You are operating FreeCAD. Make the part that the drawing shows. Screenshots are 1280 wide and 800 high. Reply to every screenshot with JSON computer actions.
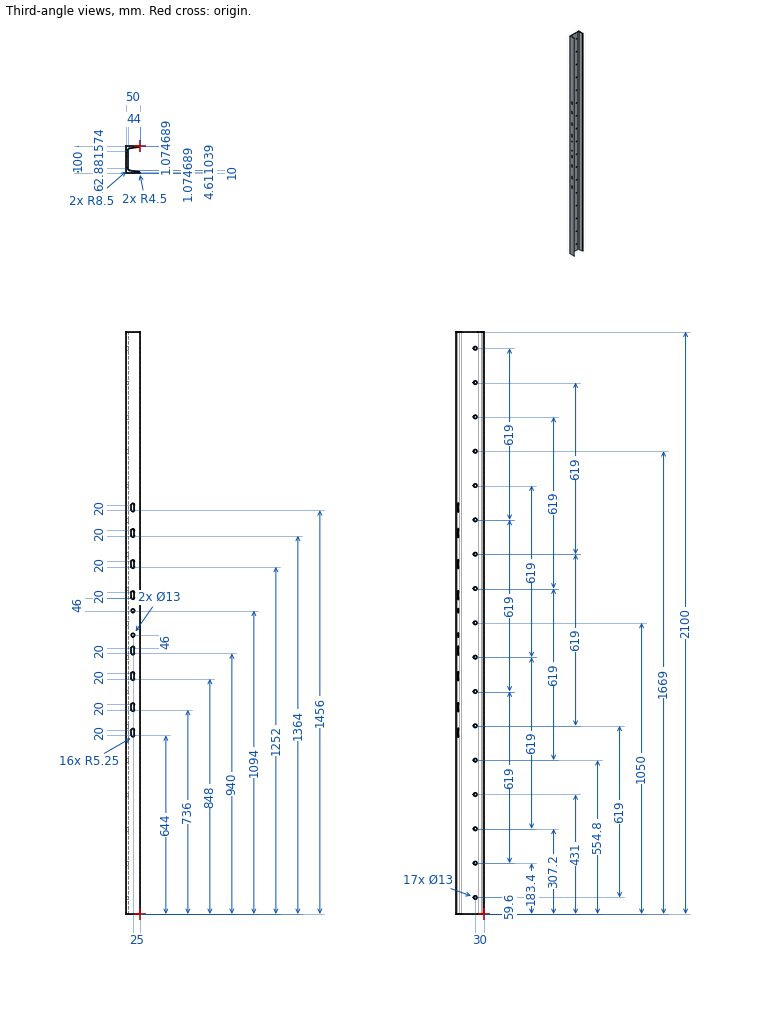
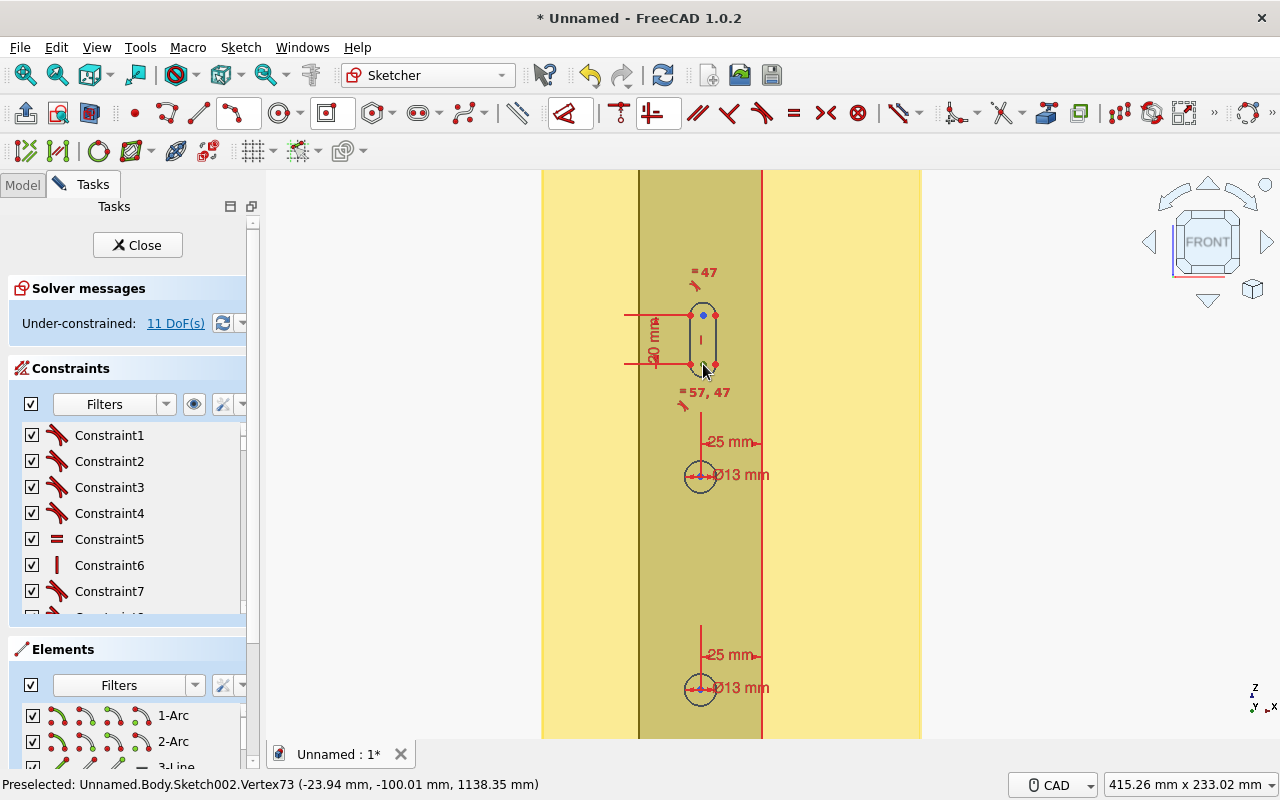
{"action": "key", "text": "l"}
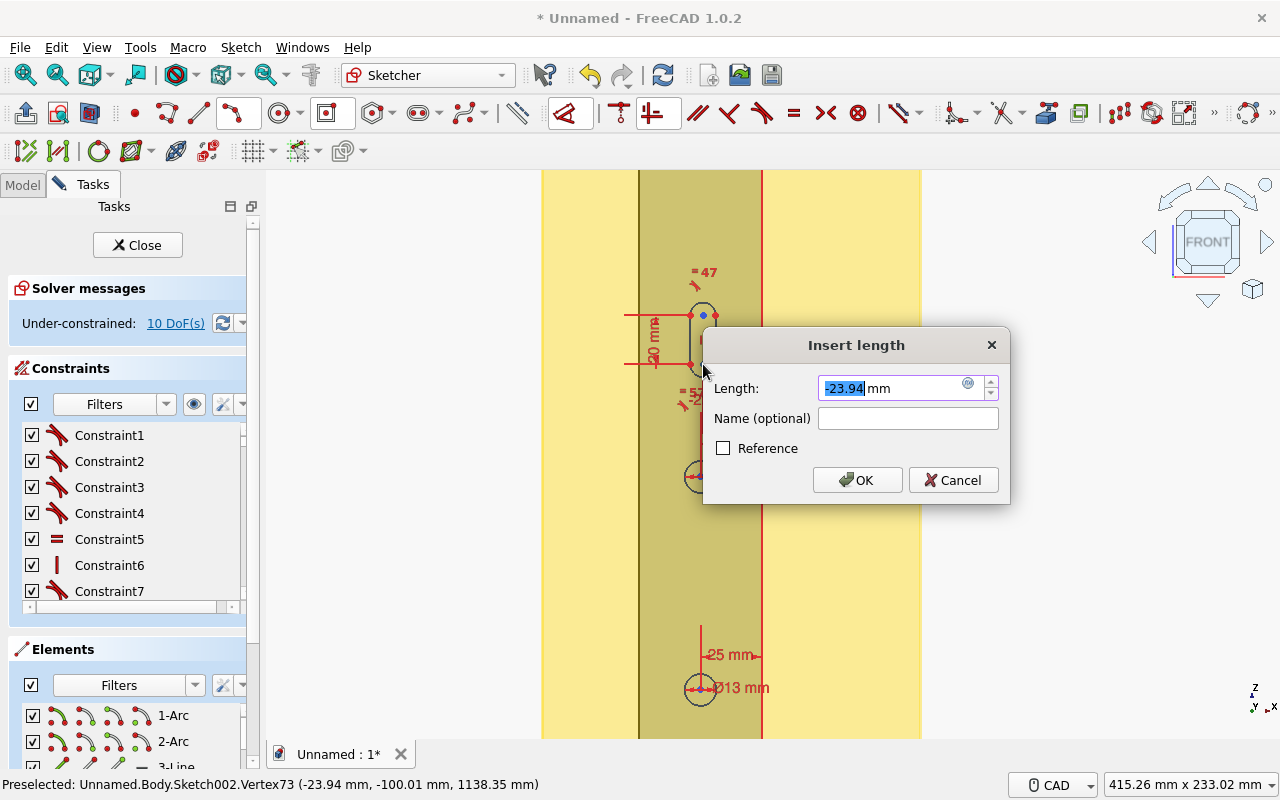
{"action": "type", "text": "-25"}
{"action": "key", "text": "Return"}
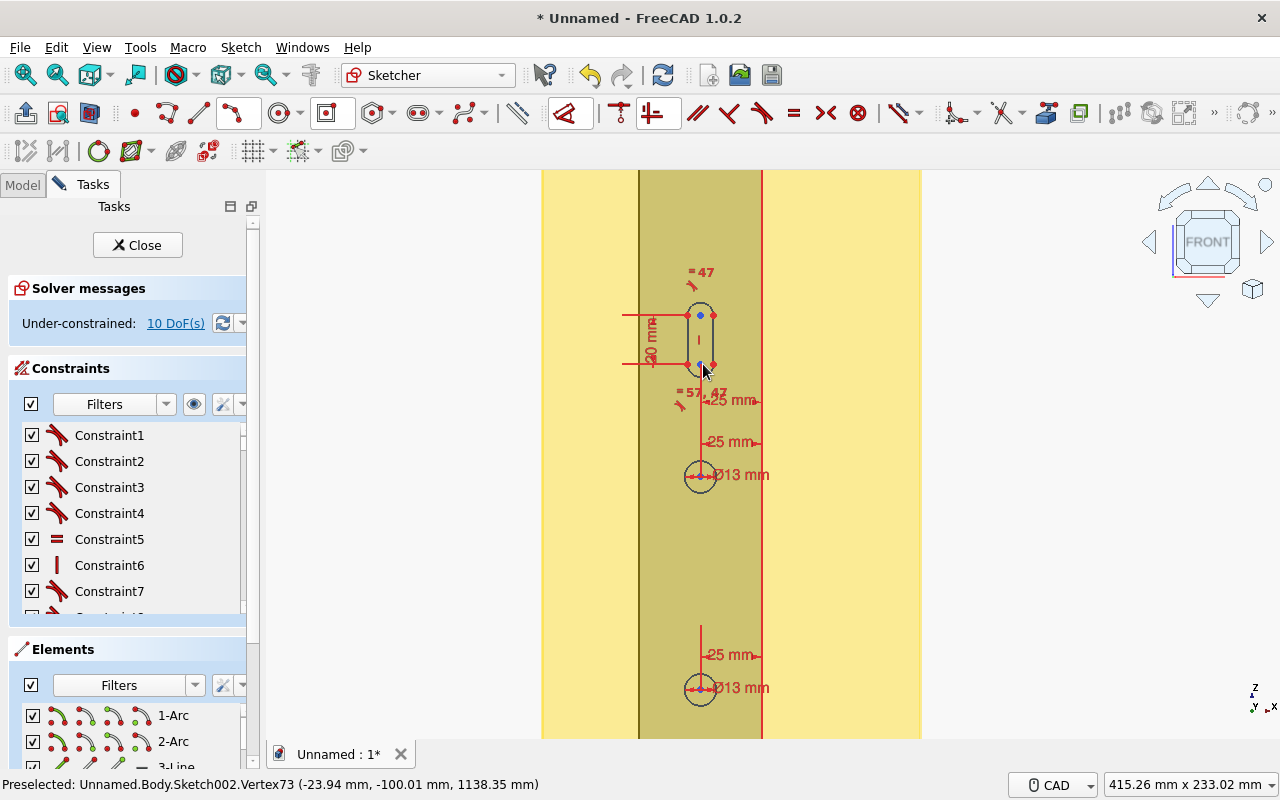
{"action": "scroll", "coordinate": [703, 367], "scroll_direction": "down", "scroll_amount": 12}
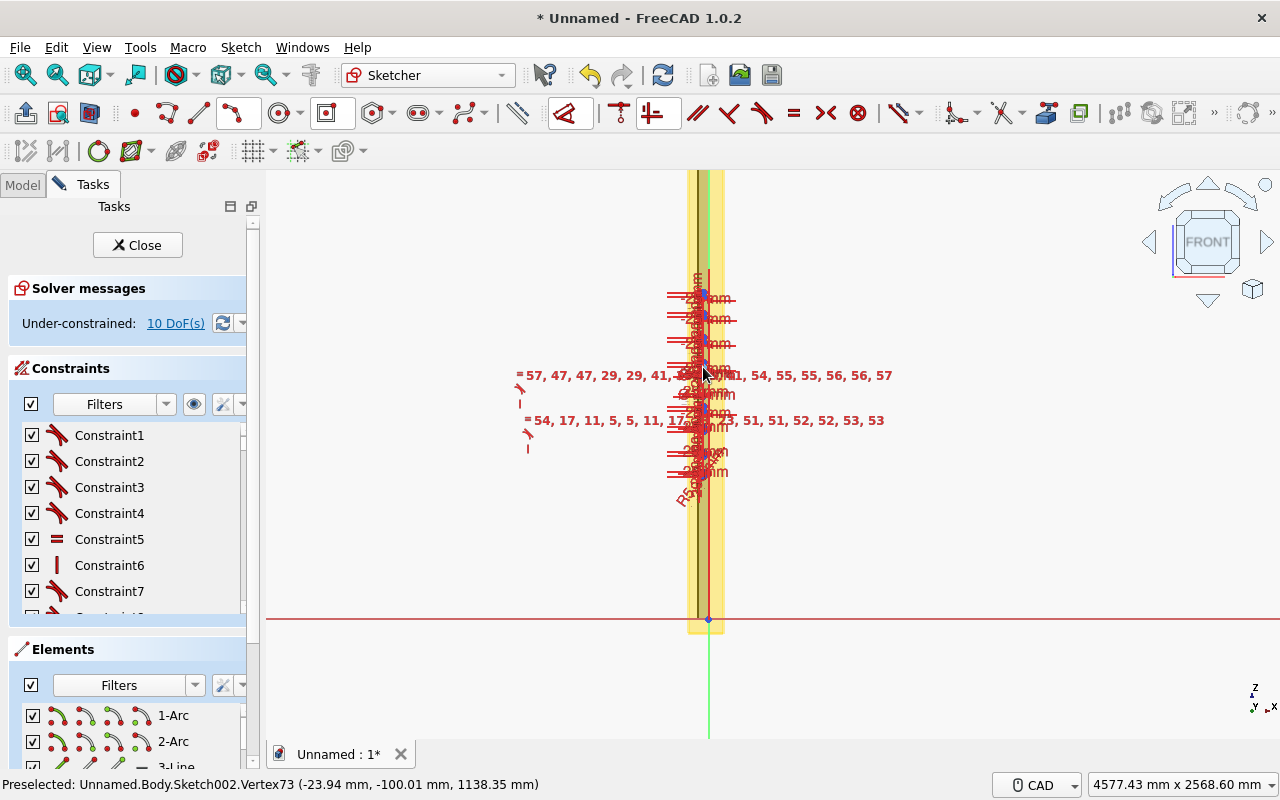
{"action": "scroll", "coordinate": [704, 407], "scroll_direction": "up", "scroll_amount": 12}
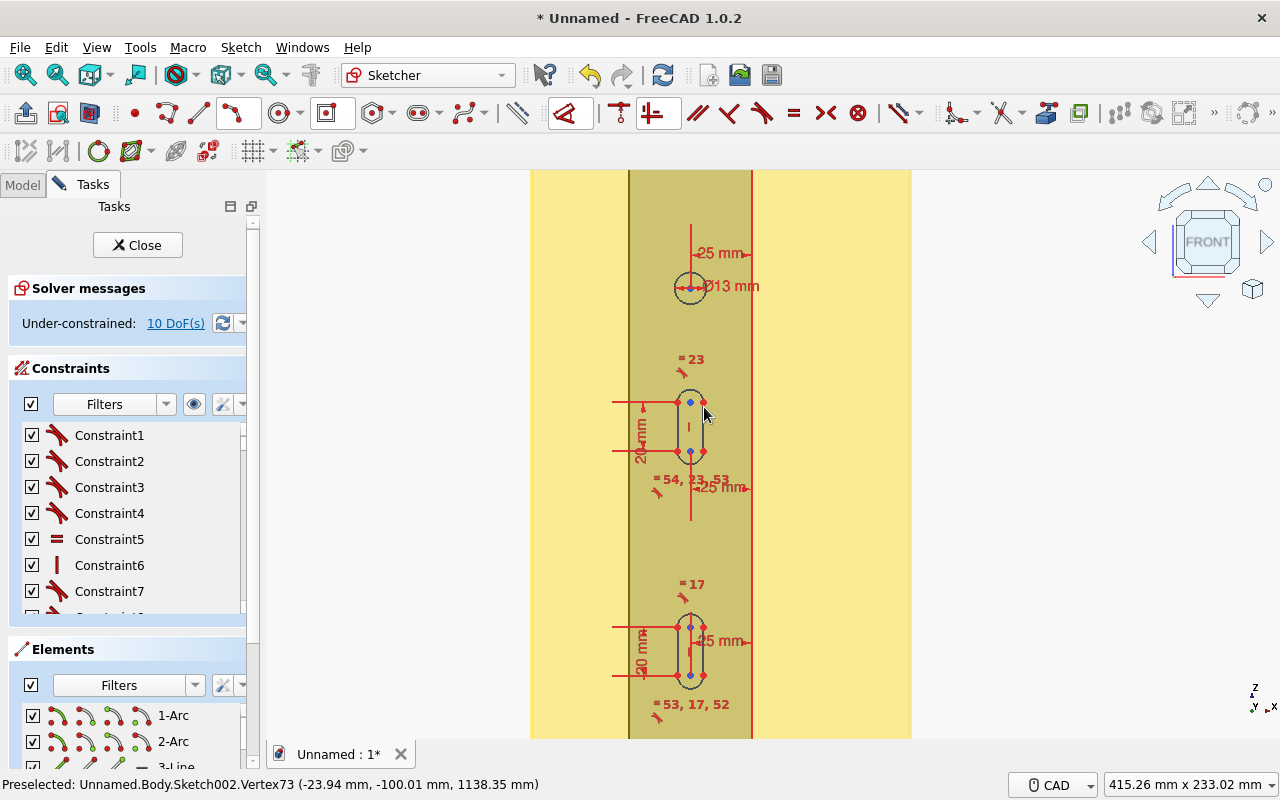
{"action": "left_click", "coordinate": [703, 402]}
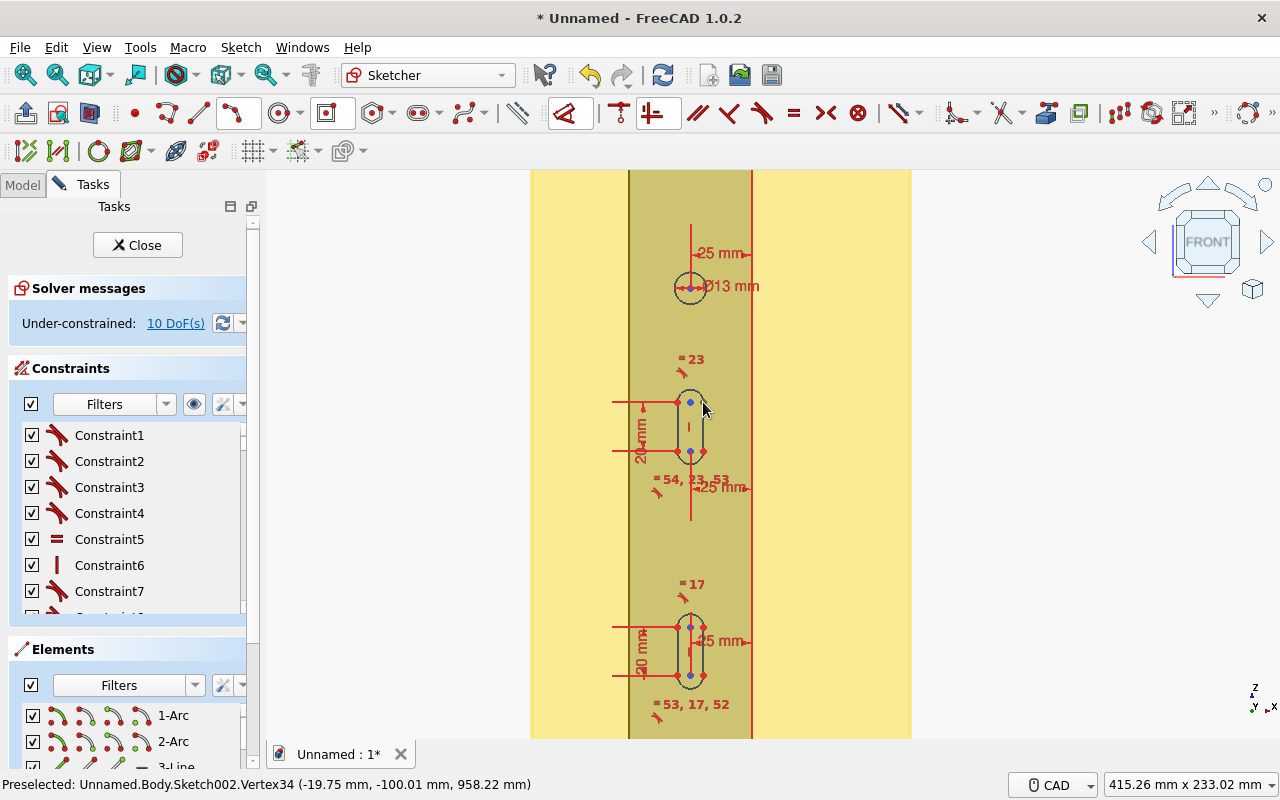
{"action": "left_click", "coordinate": [691, 288]}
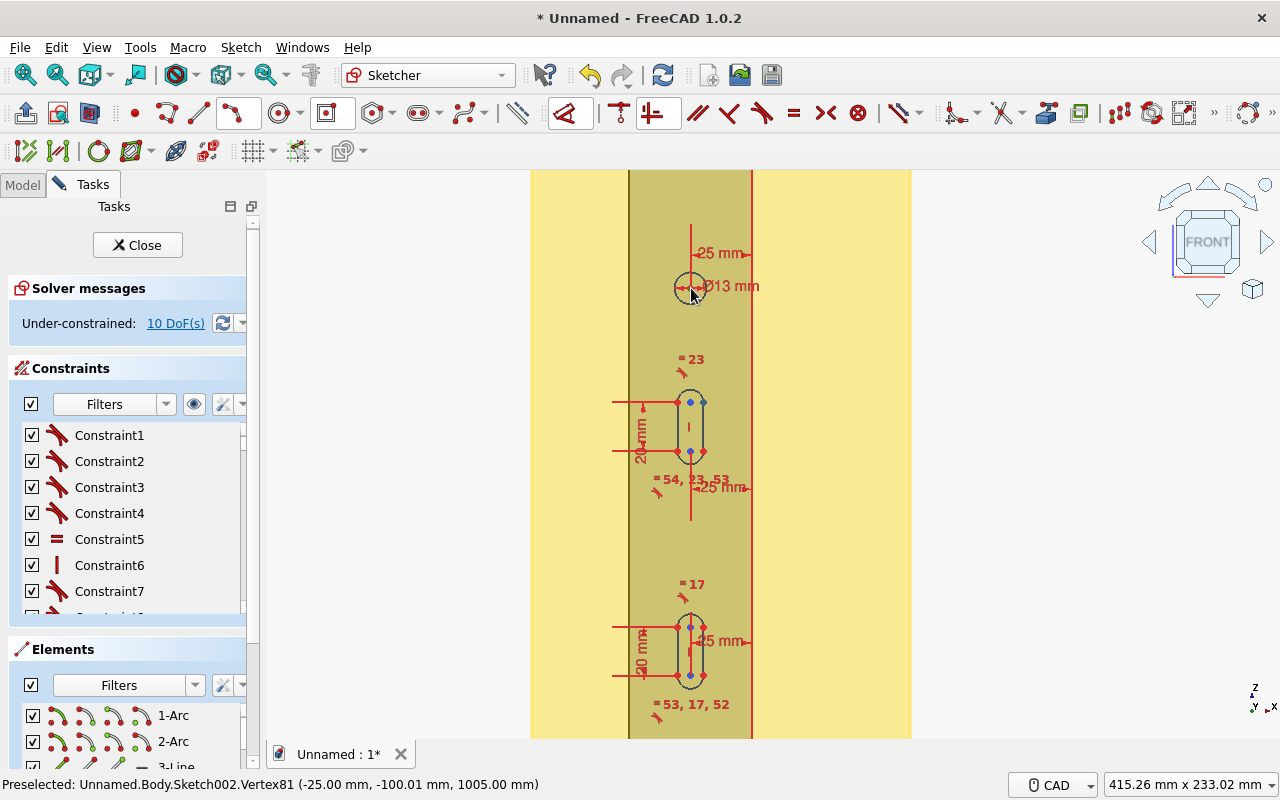
{"action": "left_click", "coordinate": [588, 114]}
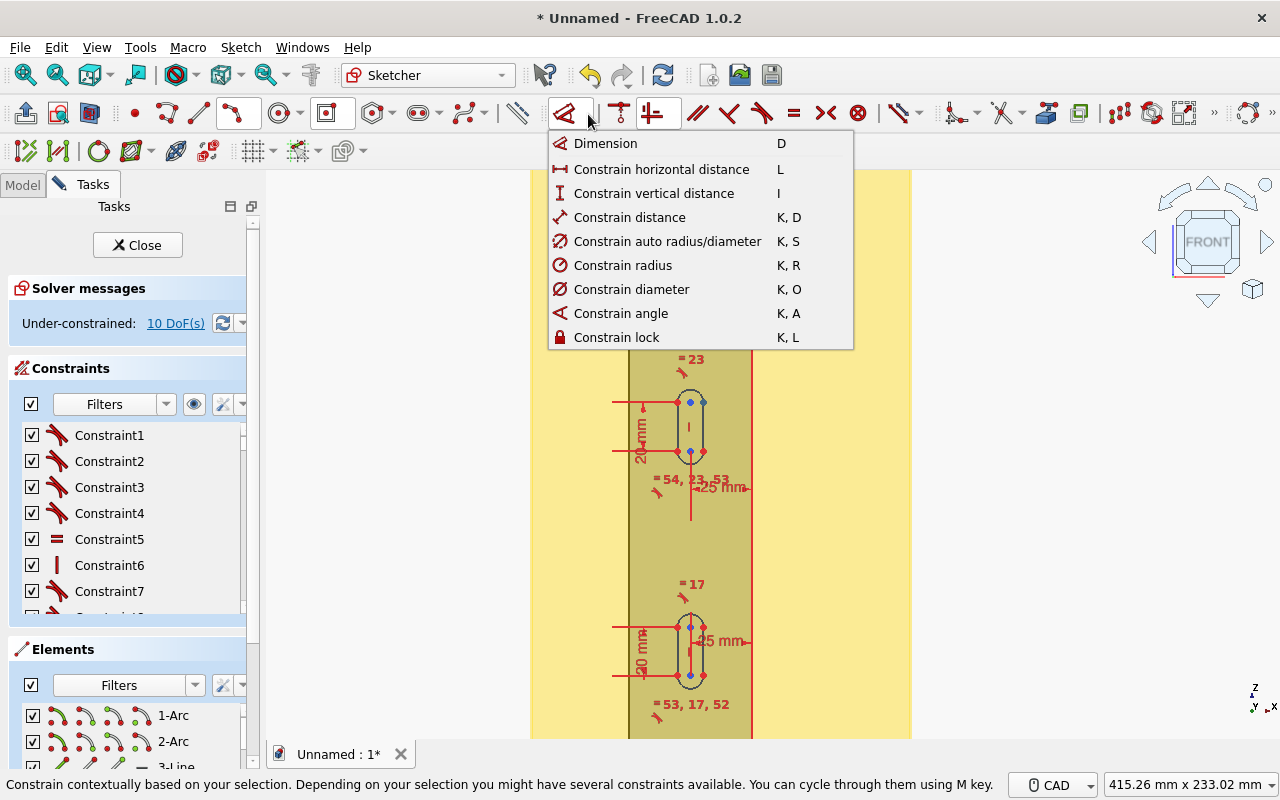
{"action": "left_click", "coordinate": [701, 193]}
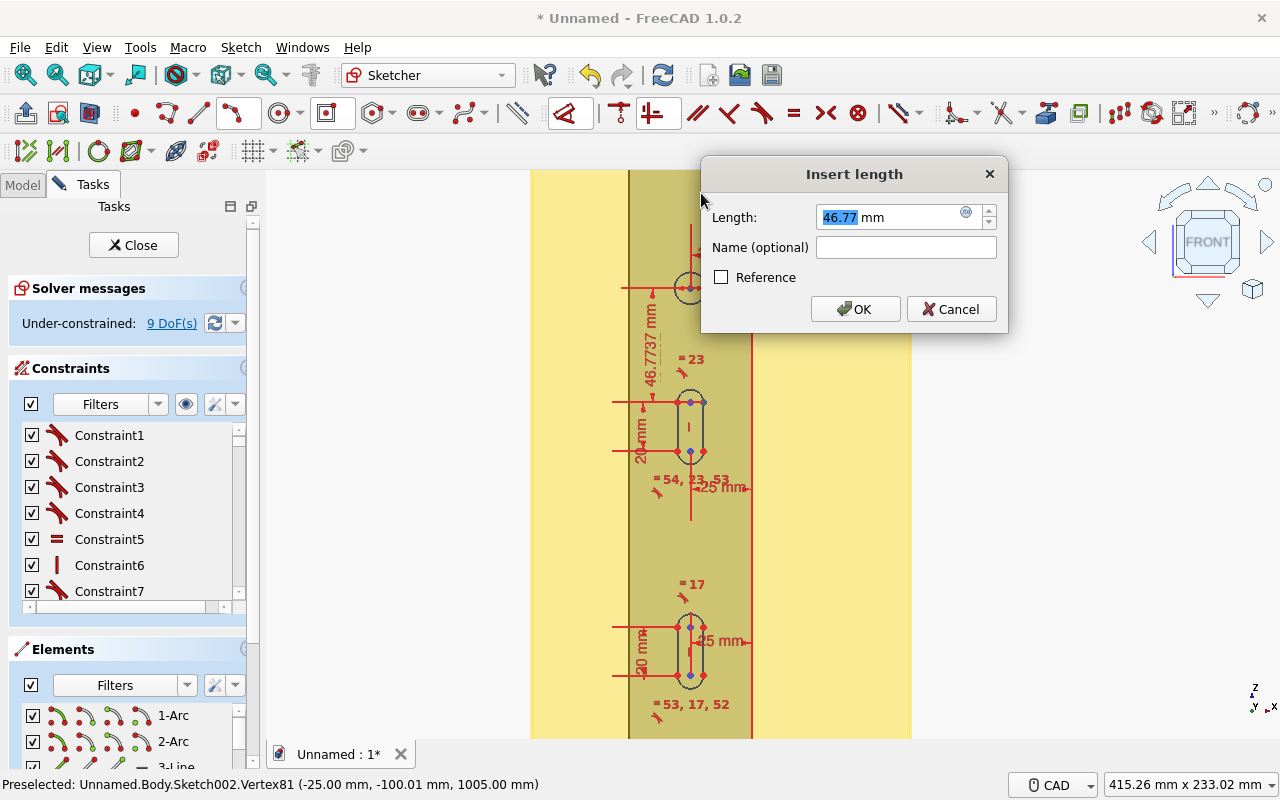
{"action": "type", "text": "46"}
{"action": "key", "text": "Return"}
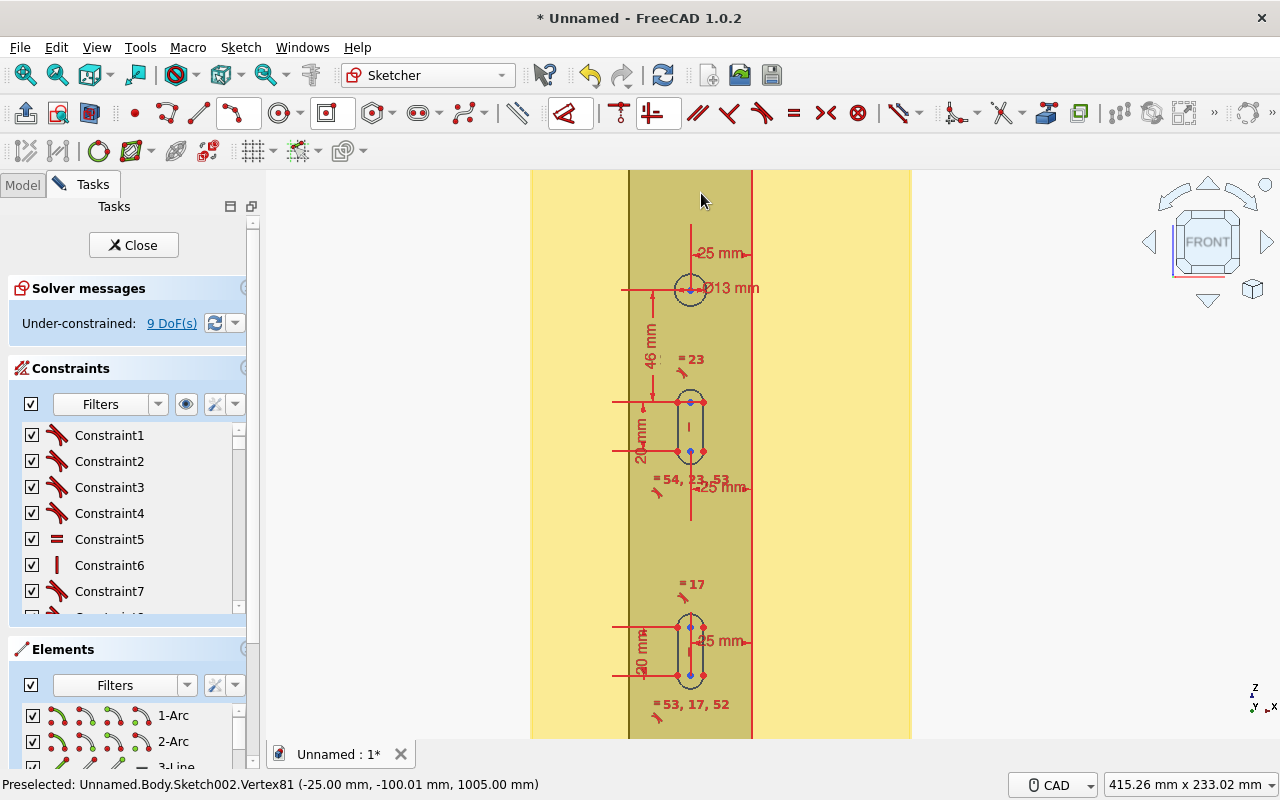
{"action": "scroll", "coordinate": [704, 407], "scroll_direction": "down", "scroll_amount": 12}